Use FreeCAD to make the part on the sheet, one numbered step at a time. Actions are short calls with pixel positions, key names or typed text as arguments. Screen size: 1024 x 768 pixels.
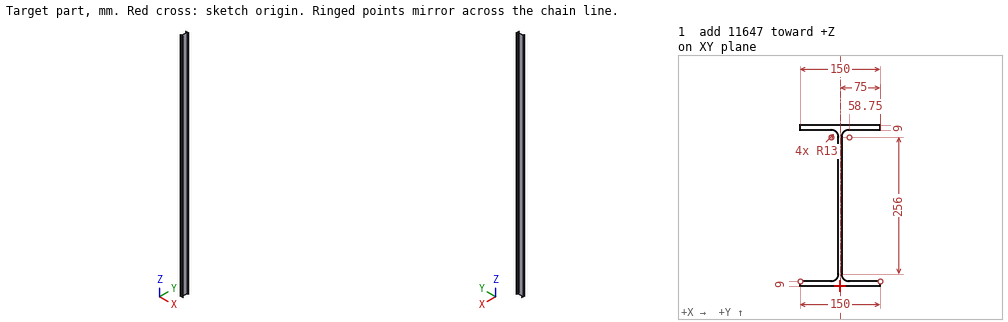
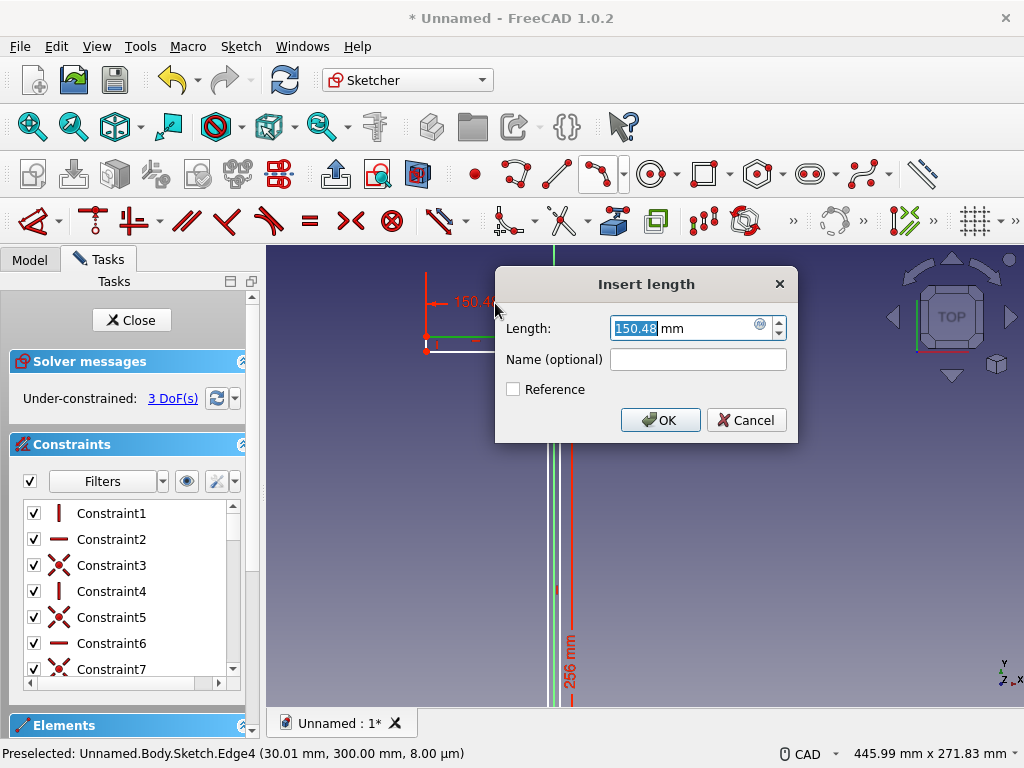
text(150)
key(Return)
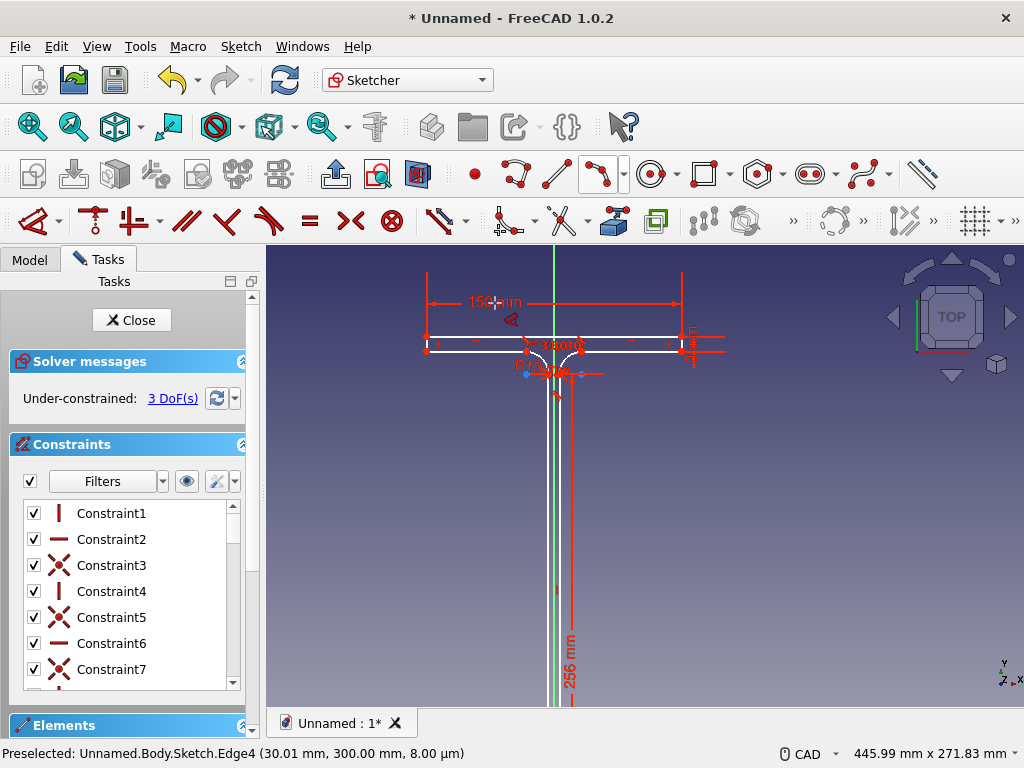
scroll(604, 335, down, 3)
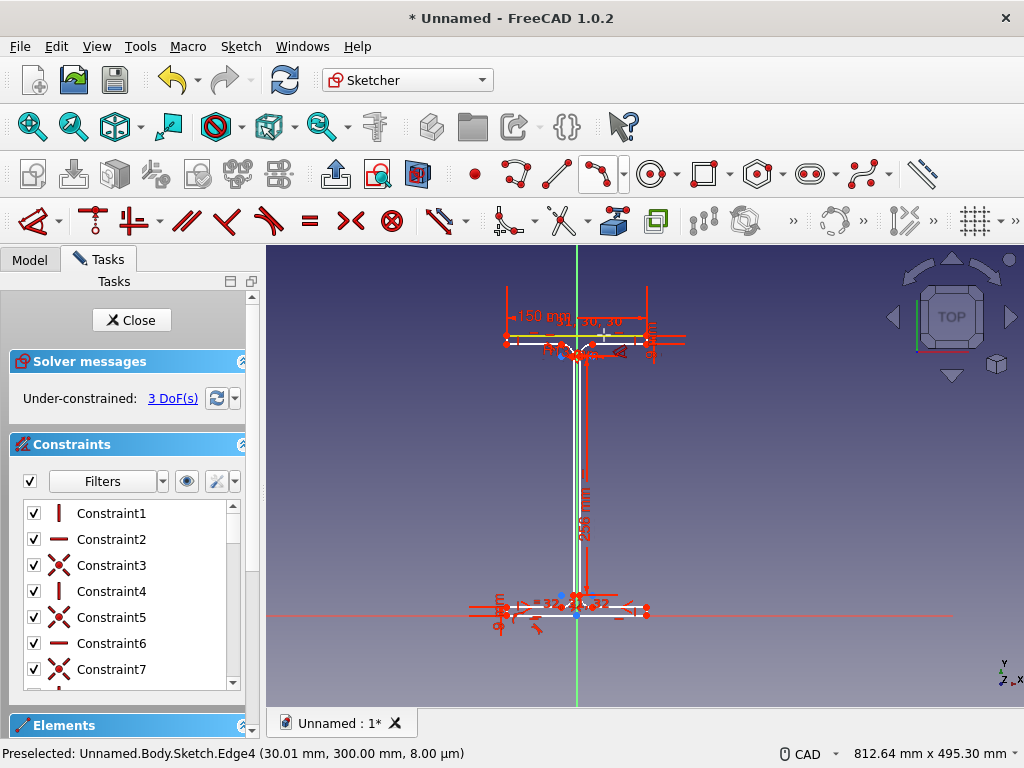
scroll(549, 616, up, 3)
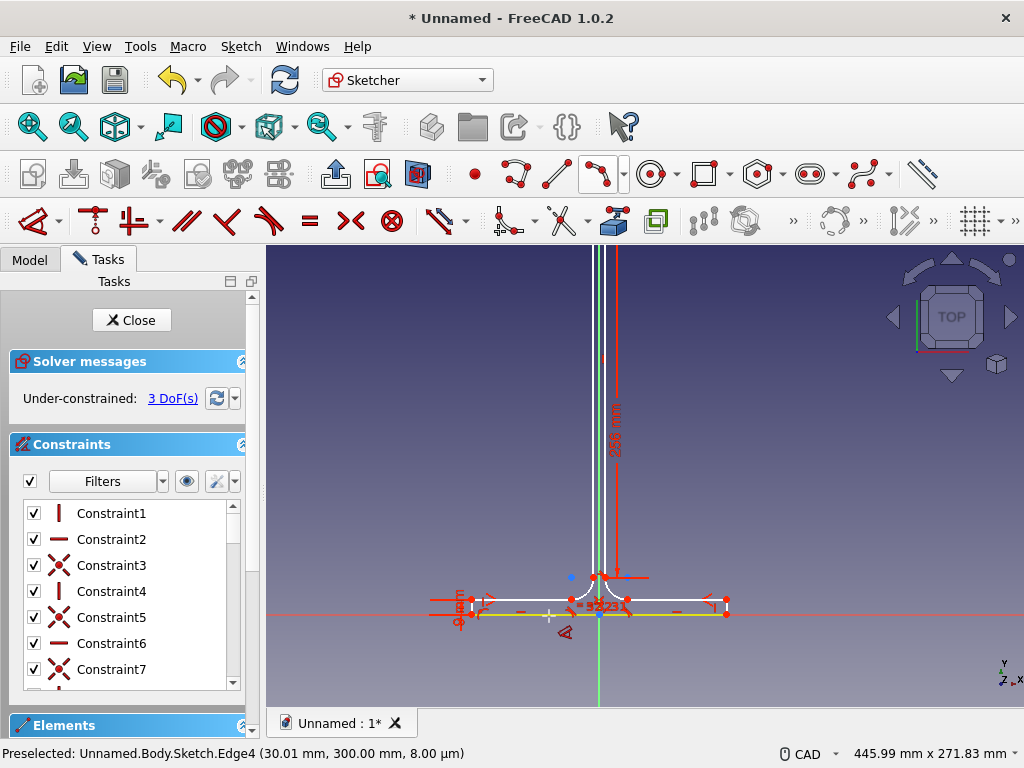
click(548, 615)
click(541, 649)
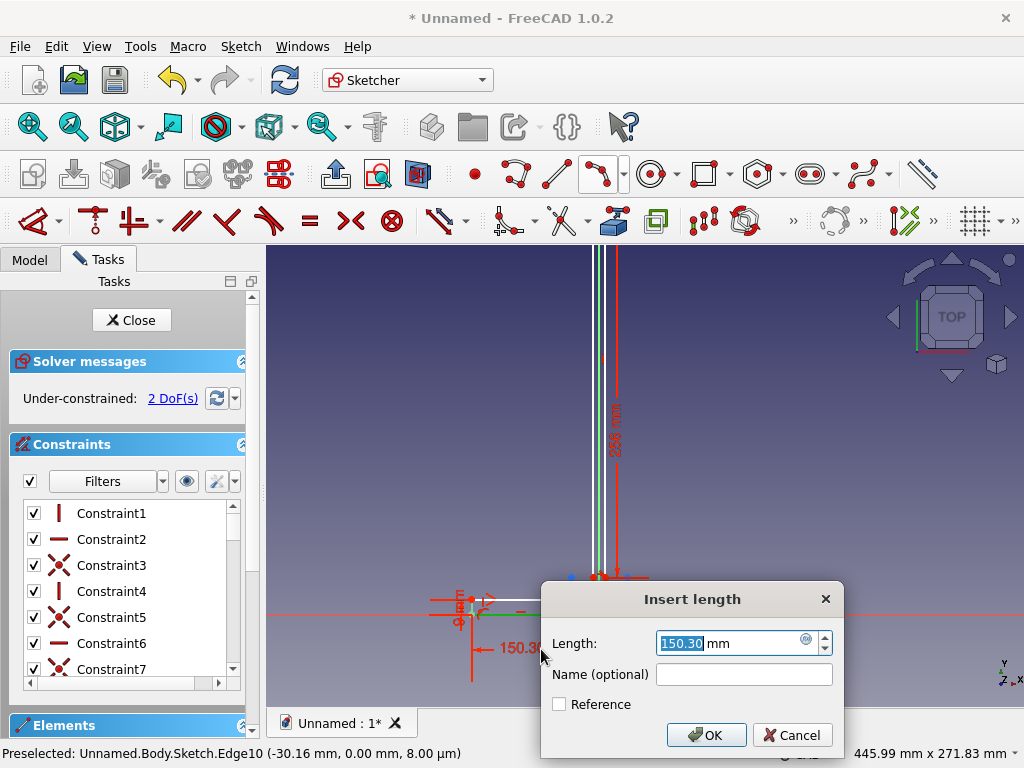
text(150)
key(Return)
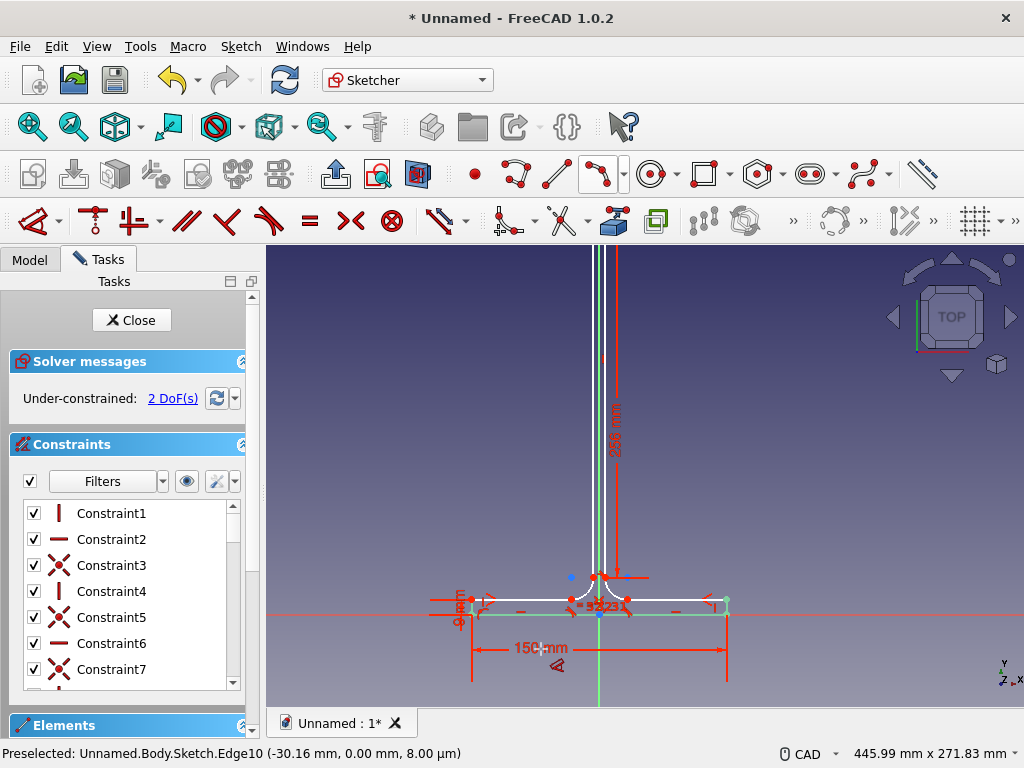
scroll(549, 617, down, 3)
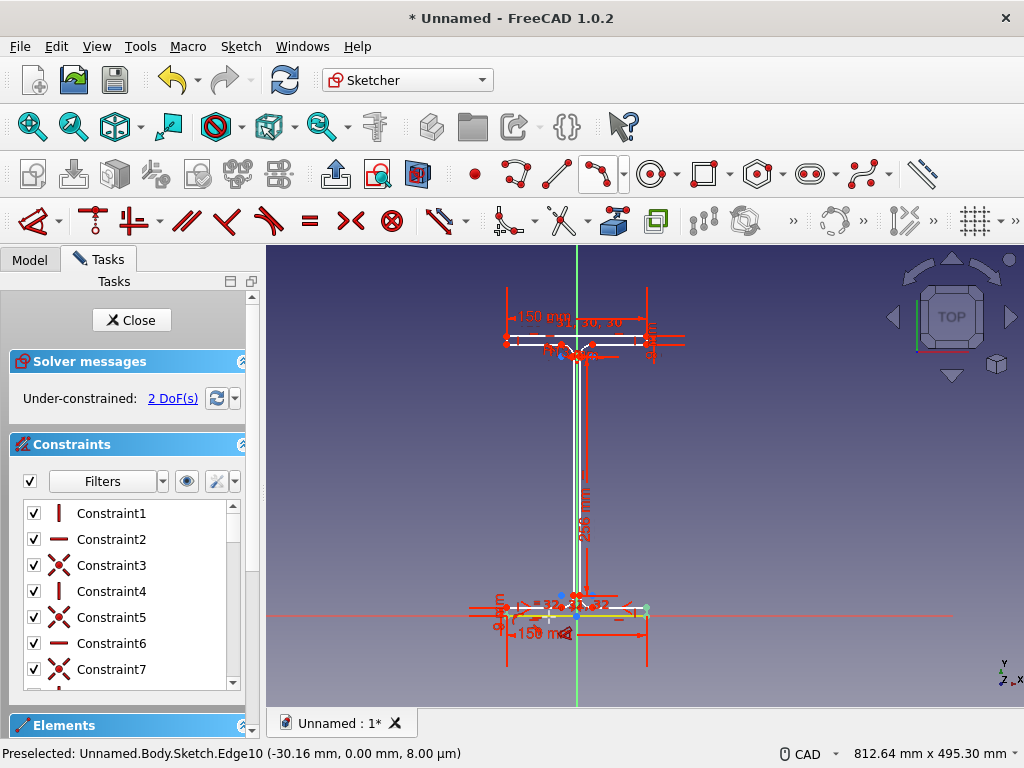
scroll(647, 345, up, 2)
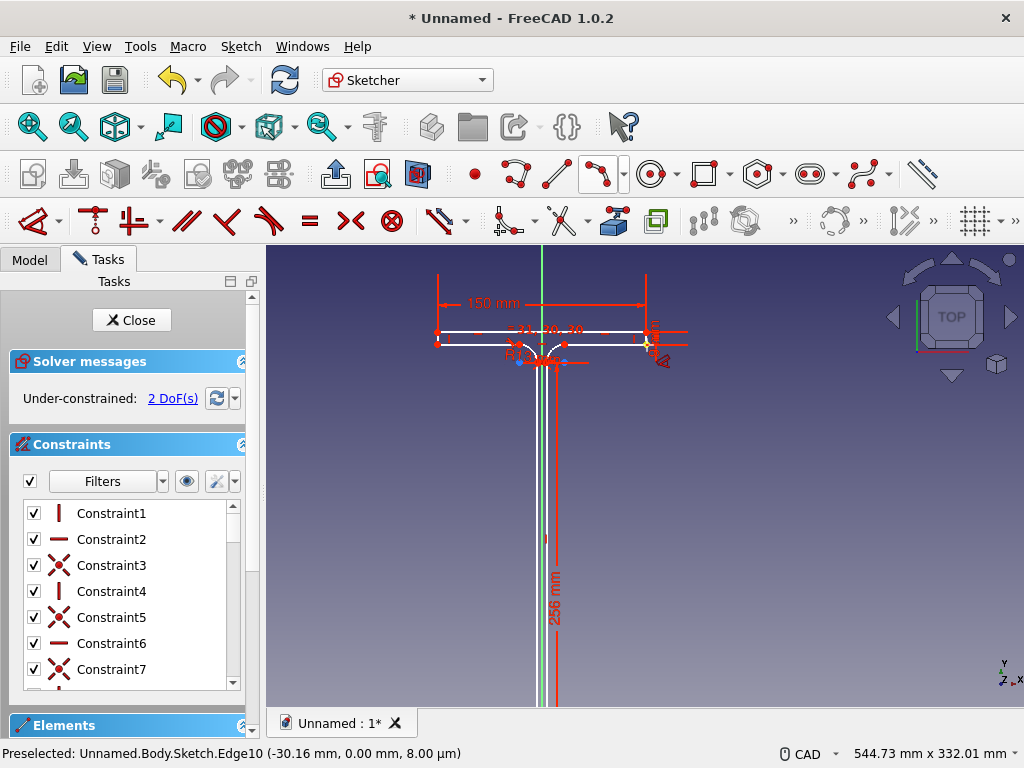
click(646, 345)
click(594, 311)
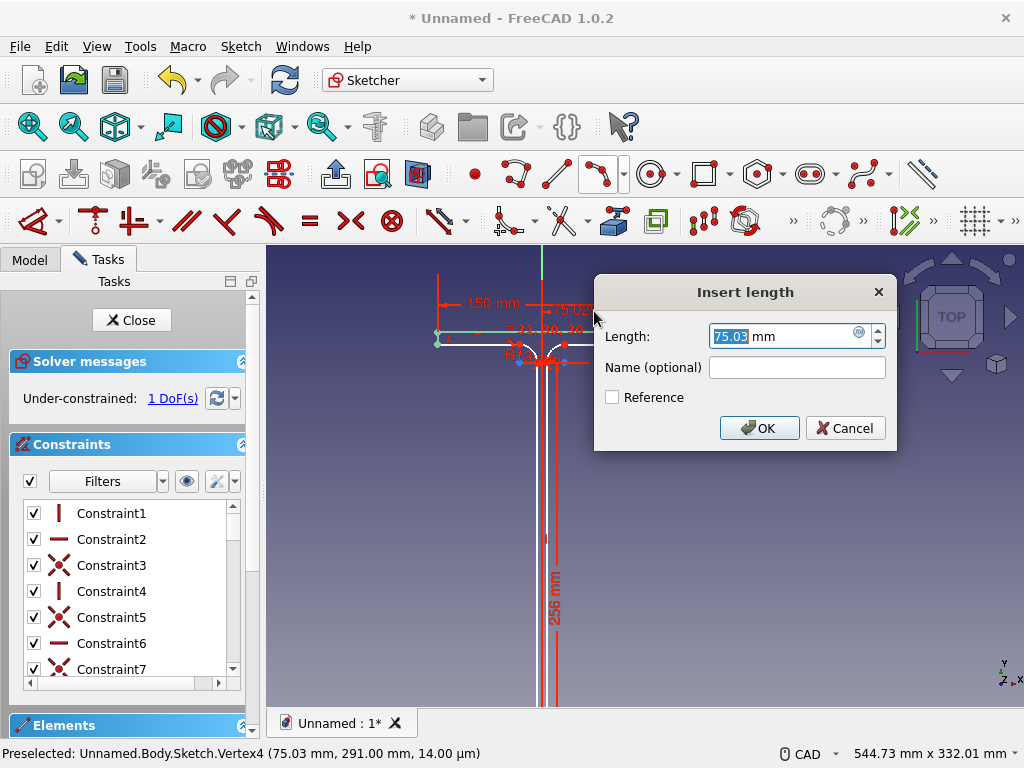
text(75)
key(Return)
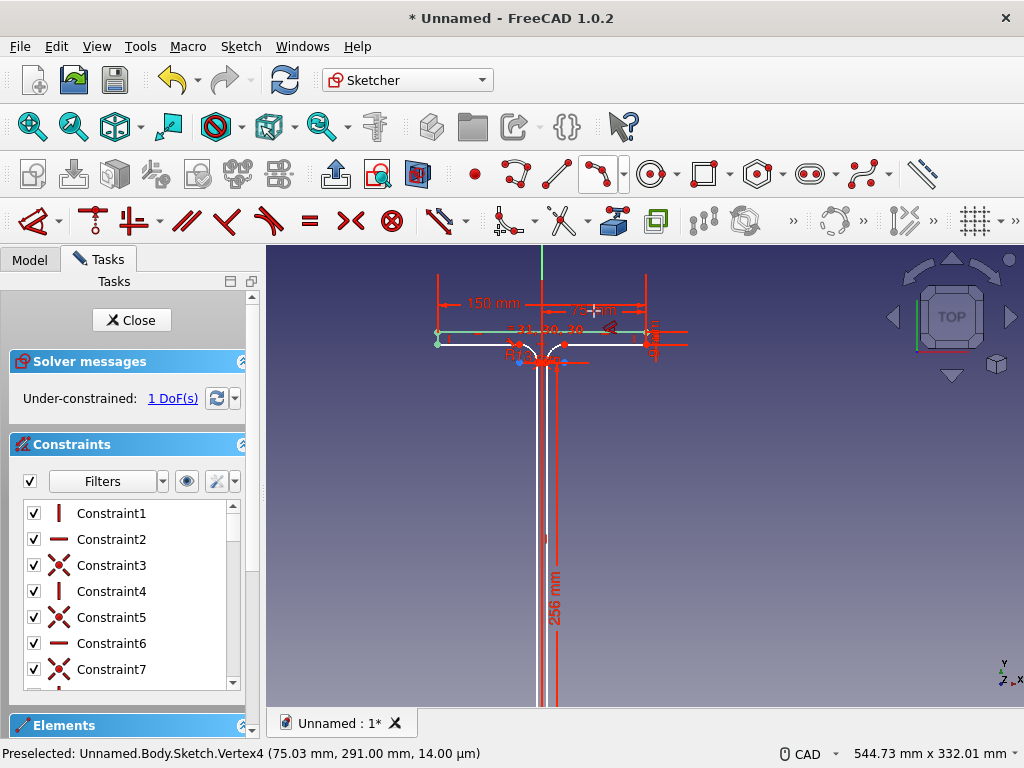
click(589, 345)
click(606, 379)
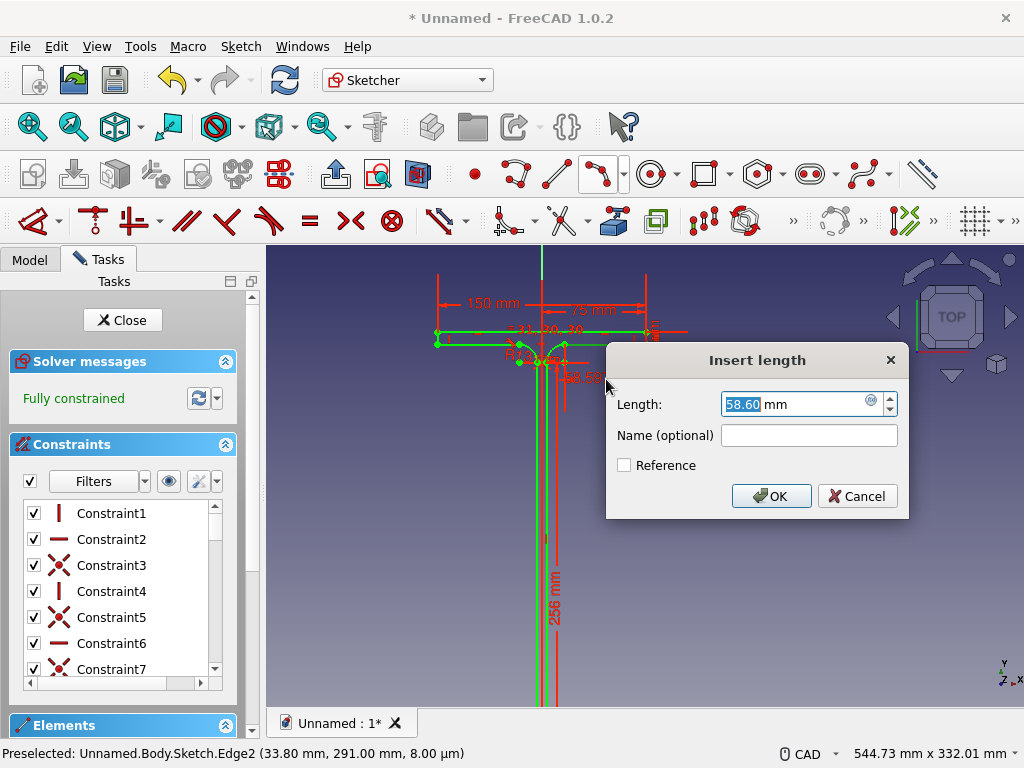
text(58.75)
key(Return)
key(Escape)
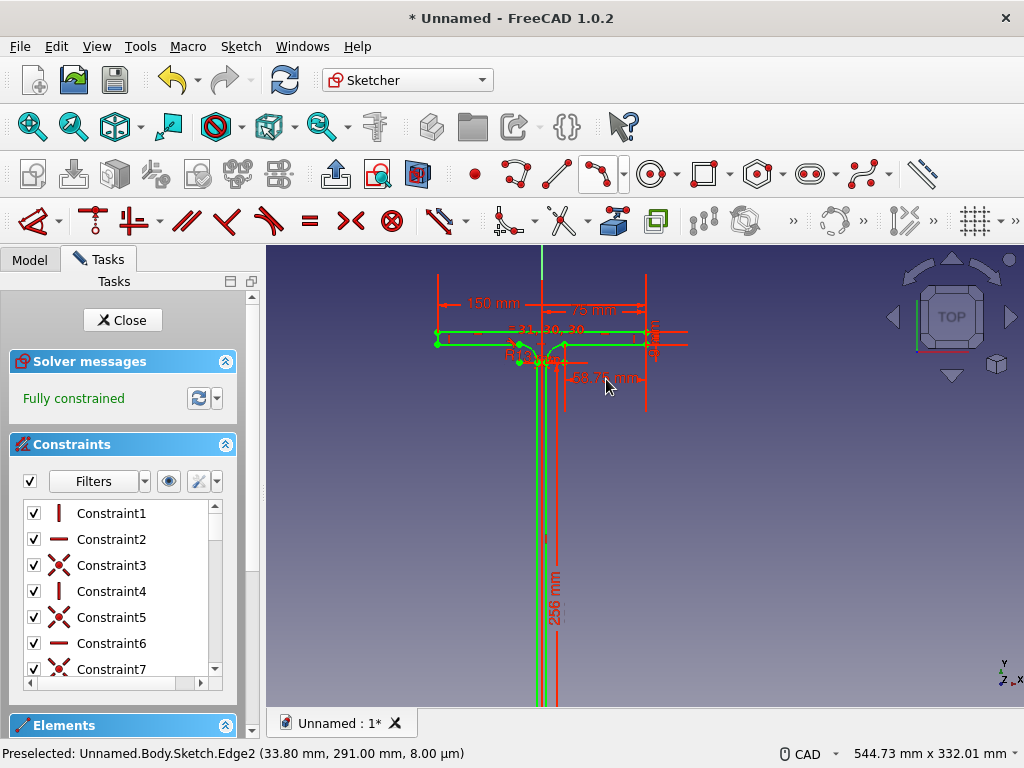
click(123, 320)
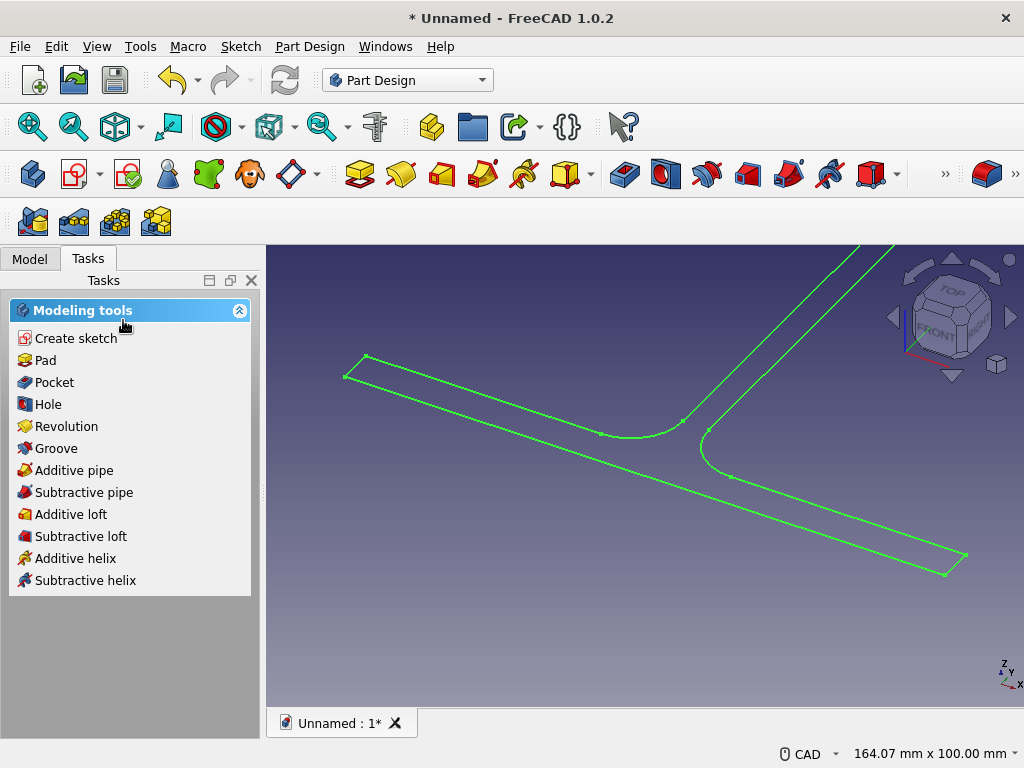
click(360, 174)